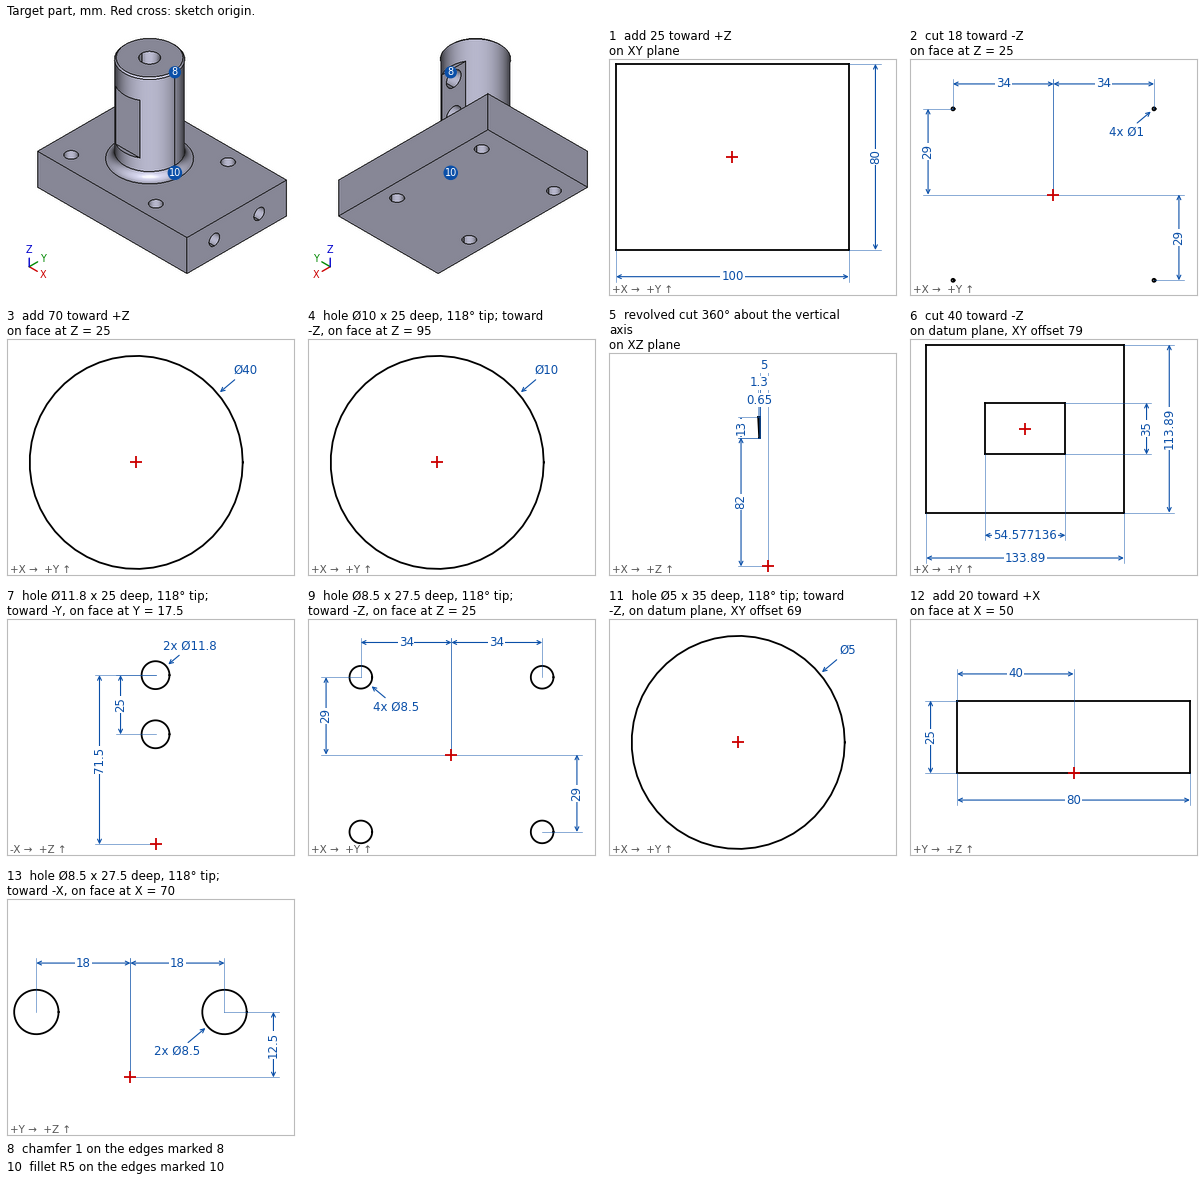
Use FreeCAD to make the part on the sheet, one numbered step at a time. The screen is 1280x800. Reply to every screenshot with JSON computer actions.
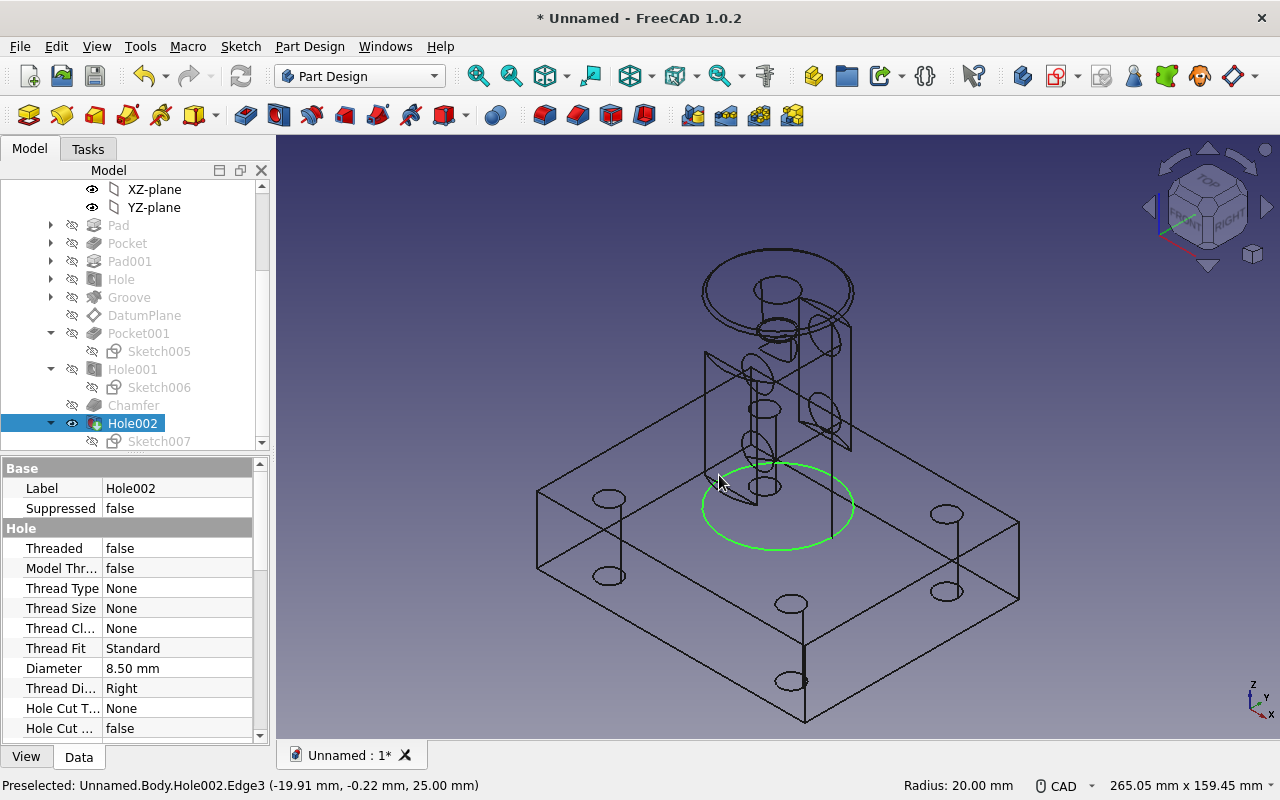
{"action": "key", "text": "v 1"}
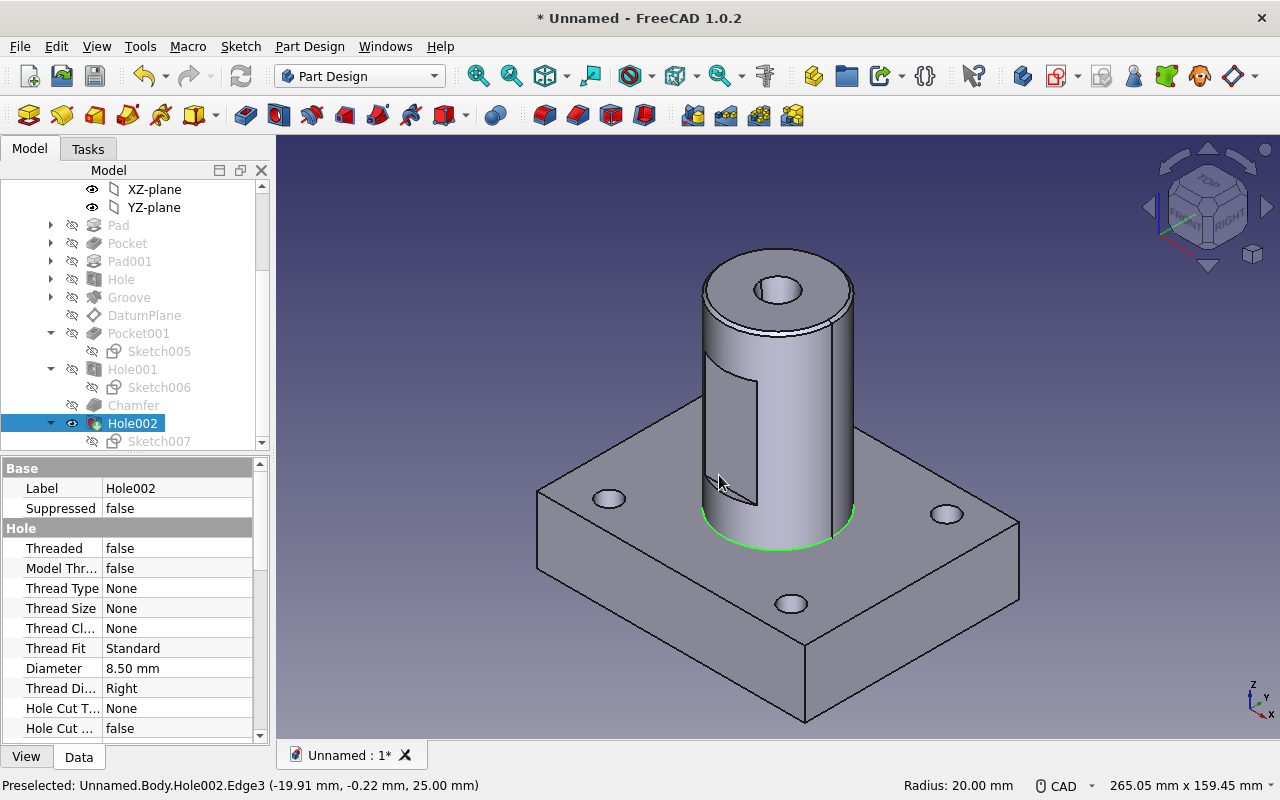
{"action": "left_click", "coordinate": [545, 116]}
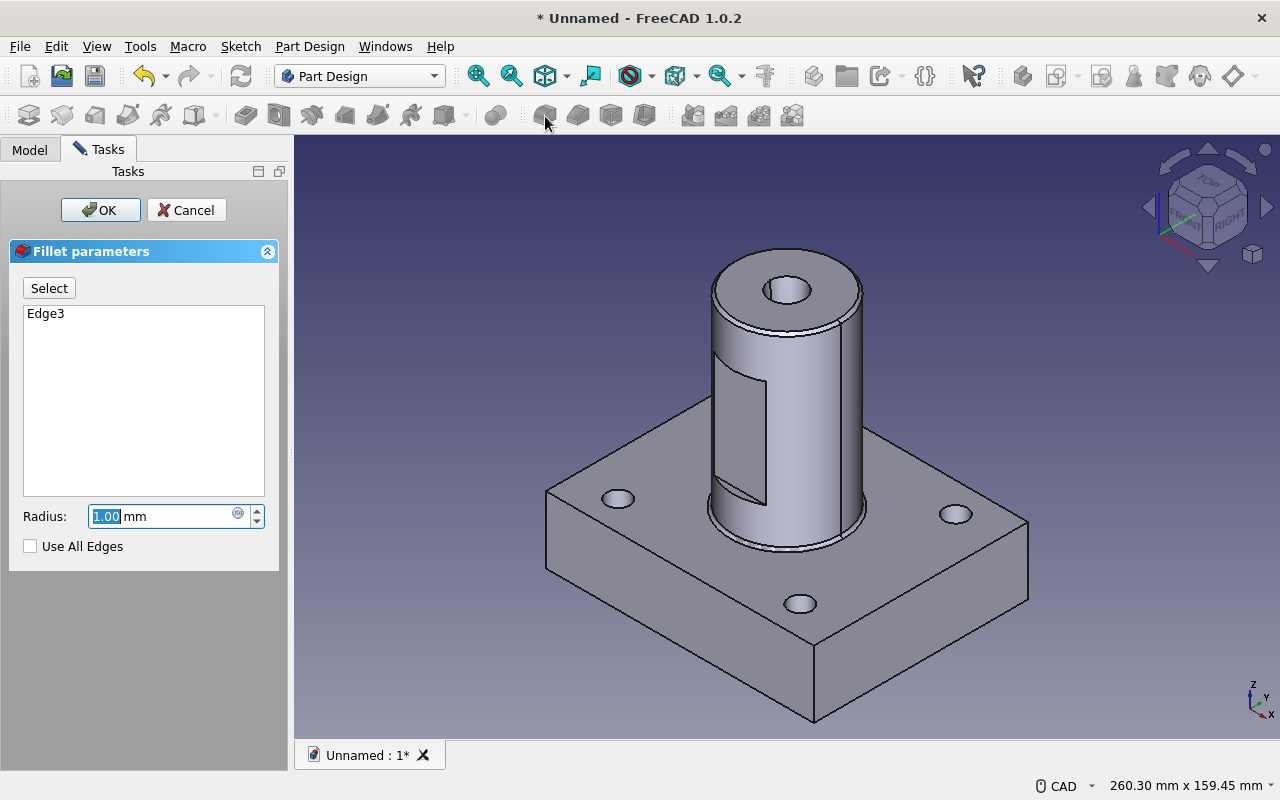
{"action": "type", "text": "5"}
{"action": "key", "text": "Tab"}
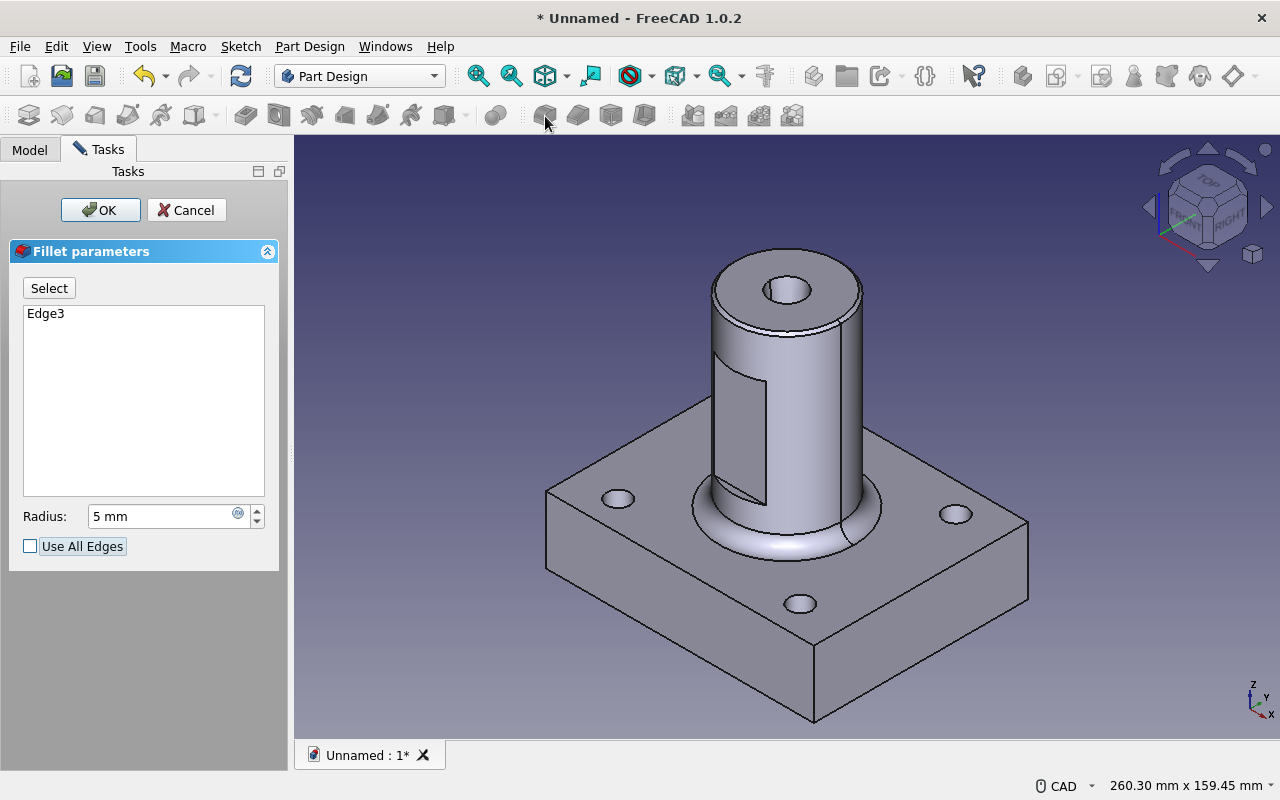
{"action": "left_click", "coordinate": [101, 210]}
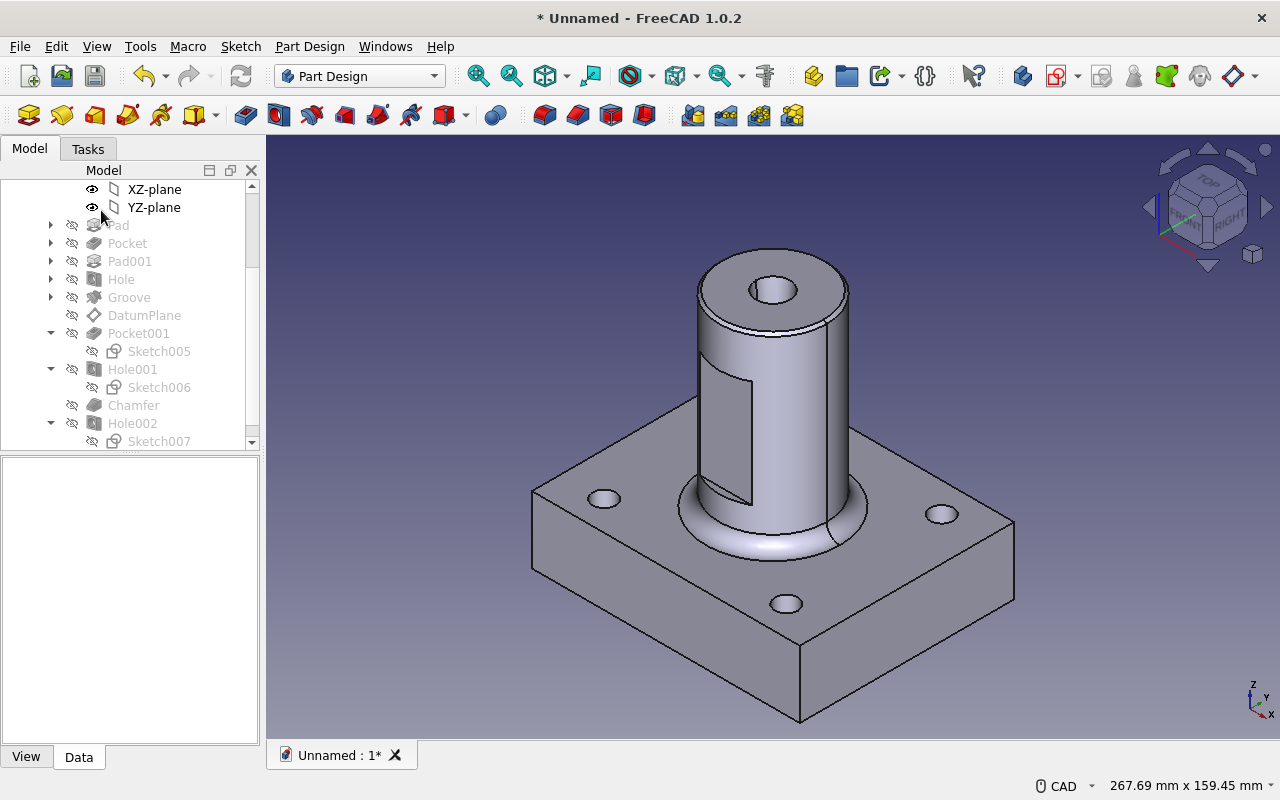
{"action": "scroll", "coordinate": [161, 311], "scroll_direction": "down", "scroll_amount": 3}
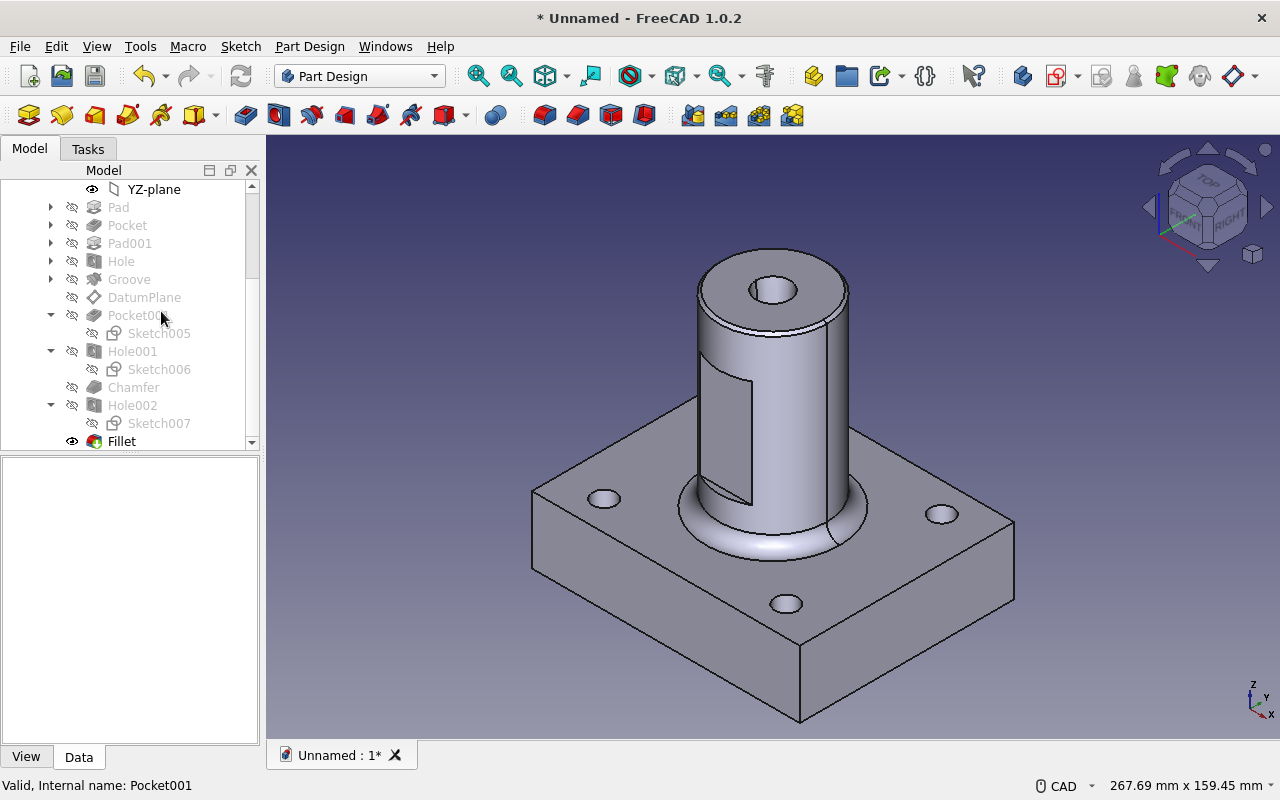
{"action": "scroll", "coordinate": [161, 311], "scroll_direction": "up", "scroll_amount": 15}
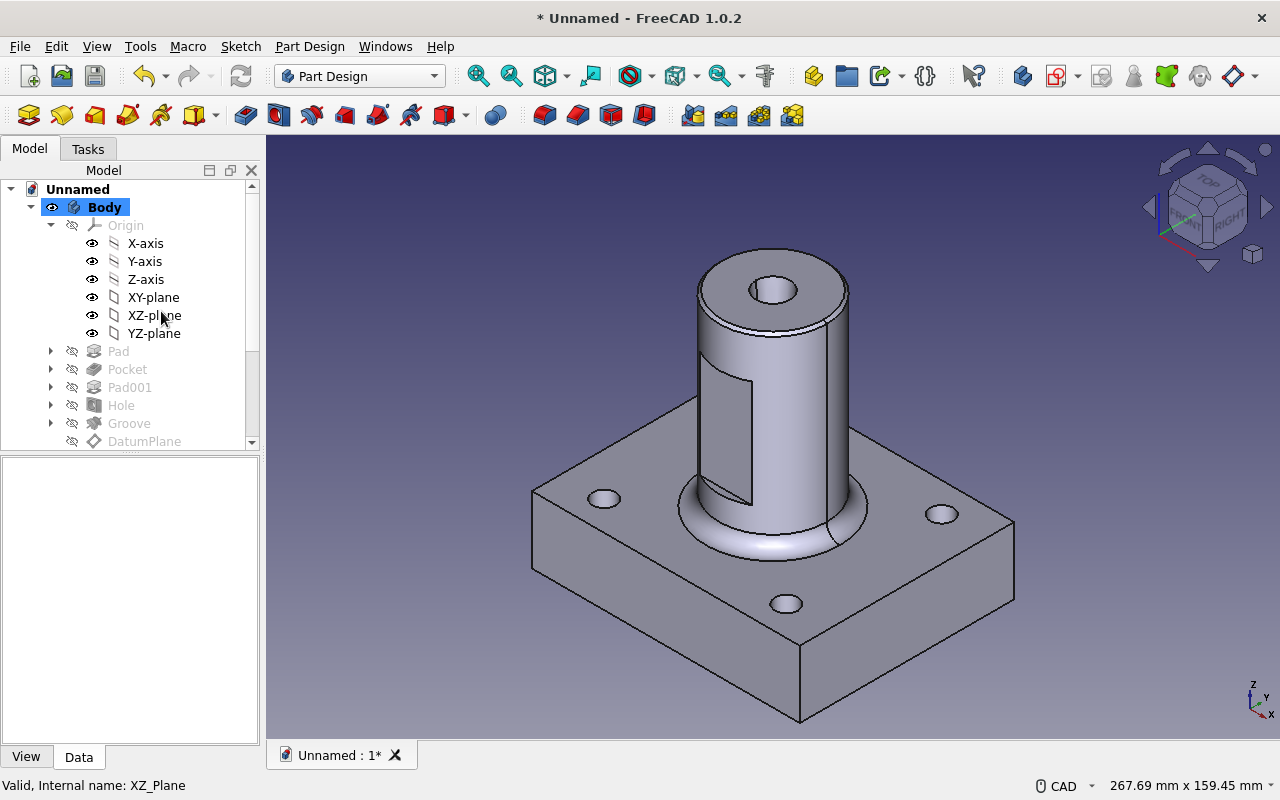
{"action": "left_click", "coordinate": [137, 297]}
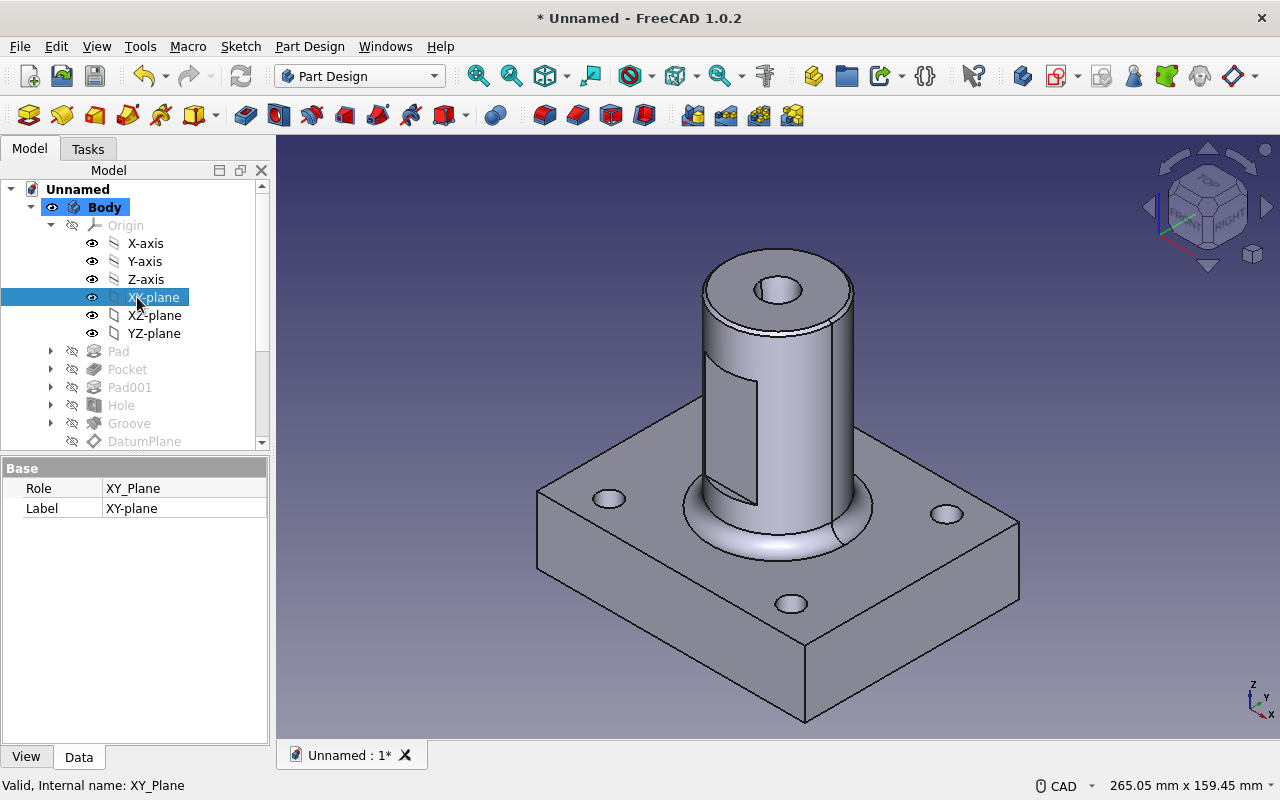
{"action": "left_click", "coordinate": [1232, 76]}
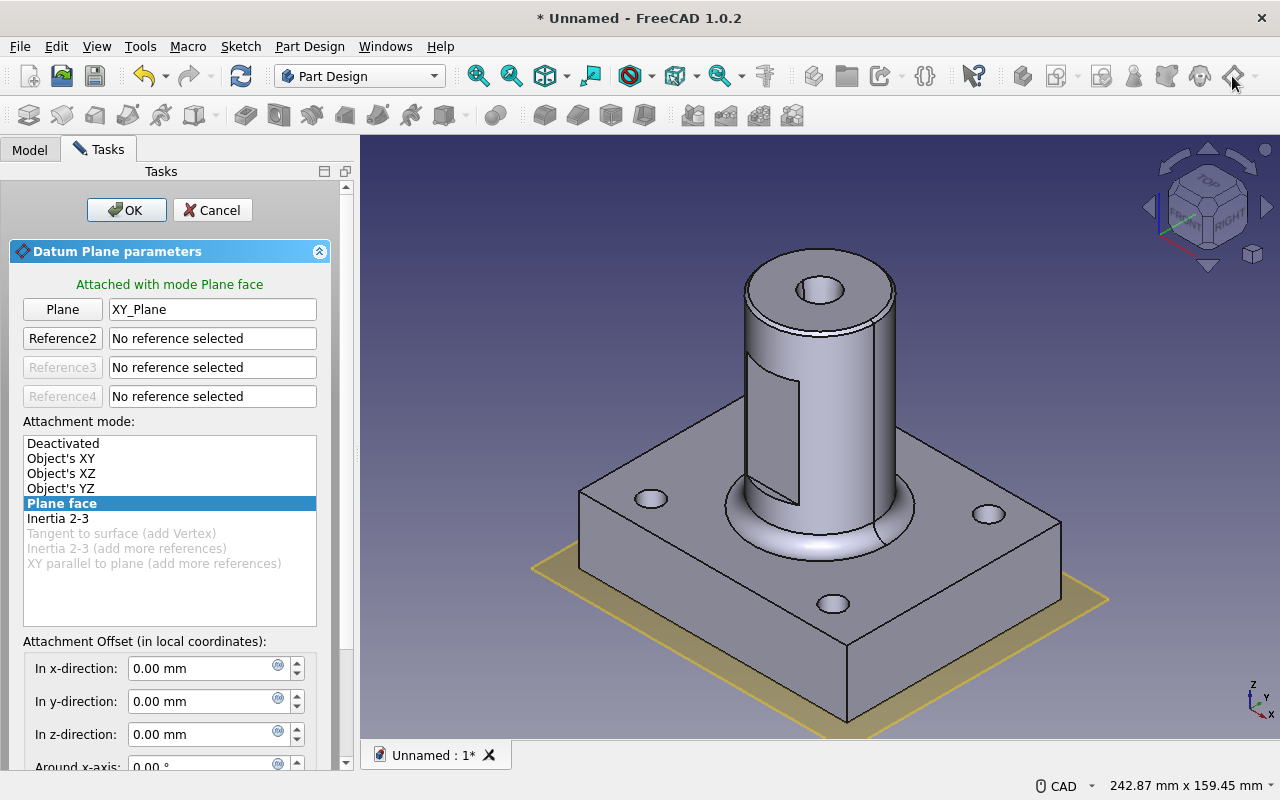
{"action": "triple_click", "coordinate": [210, 734]}